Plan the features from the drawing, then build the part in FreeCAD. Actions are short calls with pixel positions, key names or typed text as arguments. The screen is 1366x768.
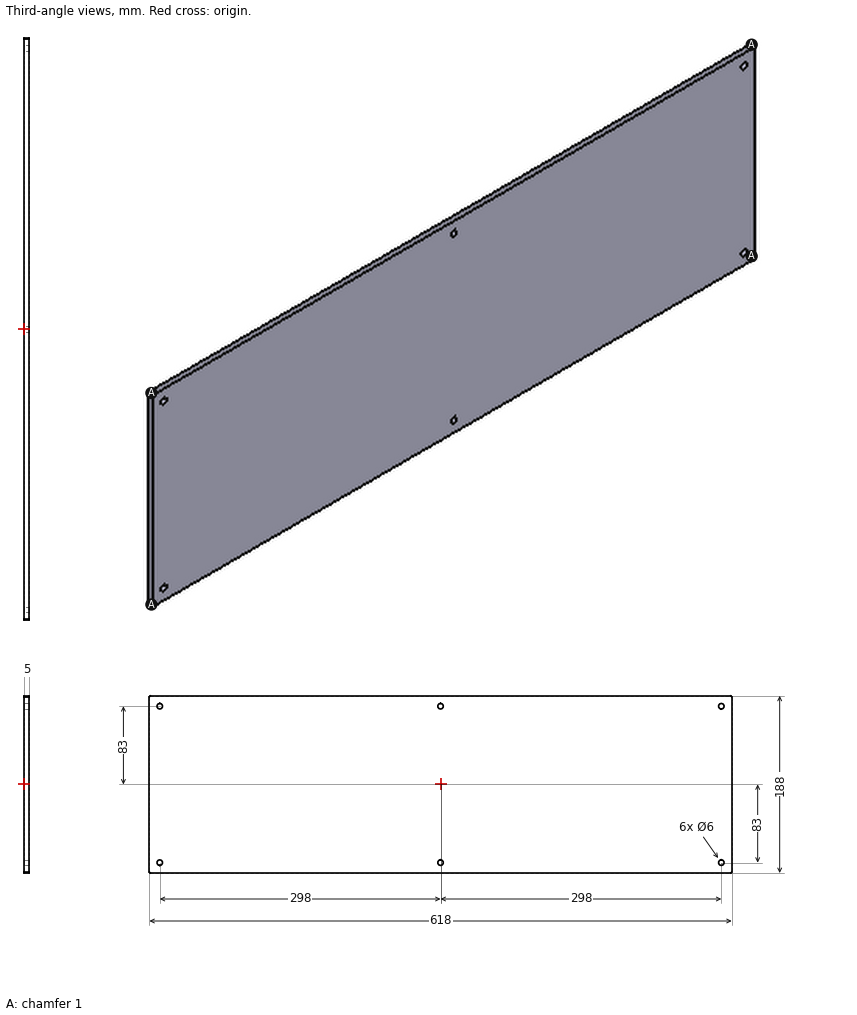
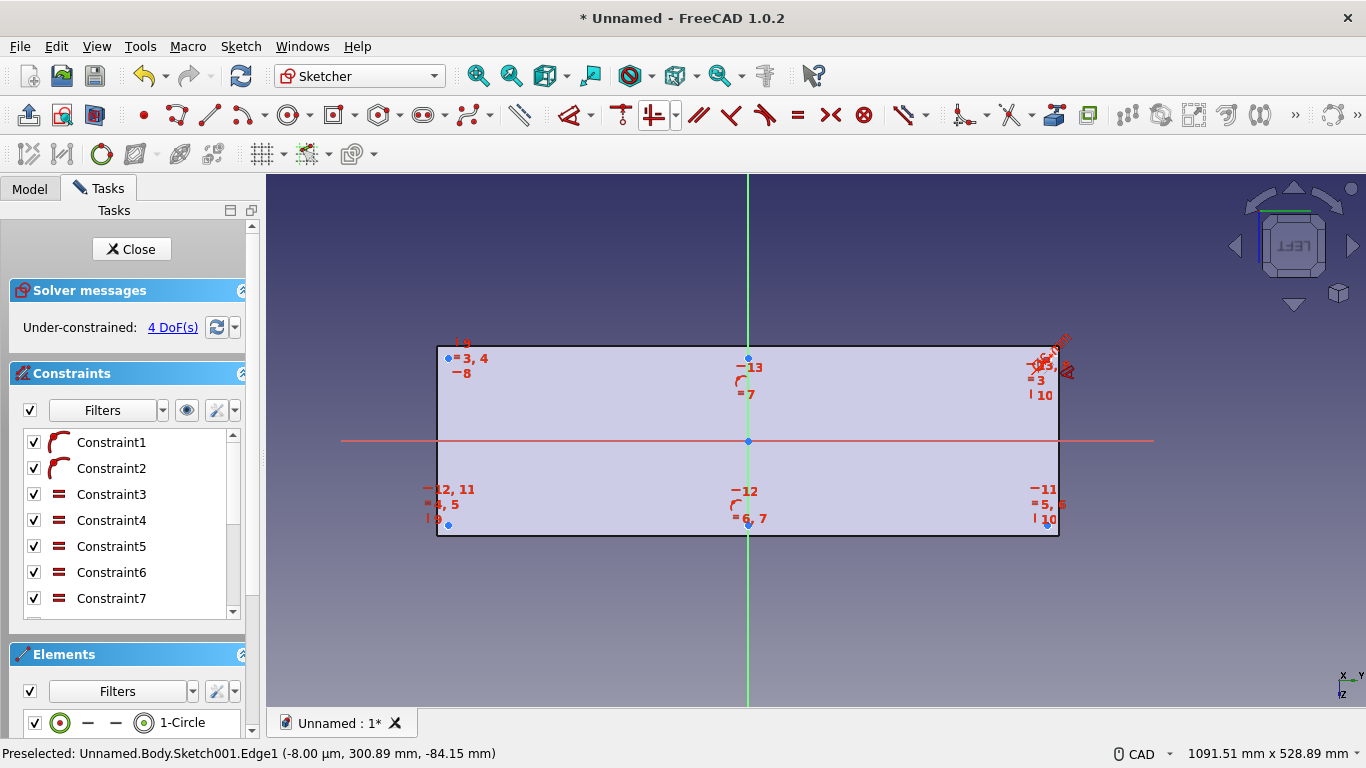
click(1048, 359)
click(1082, 400)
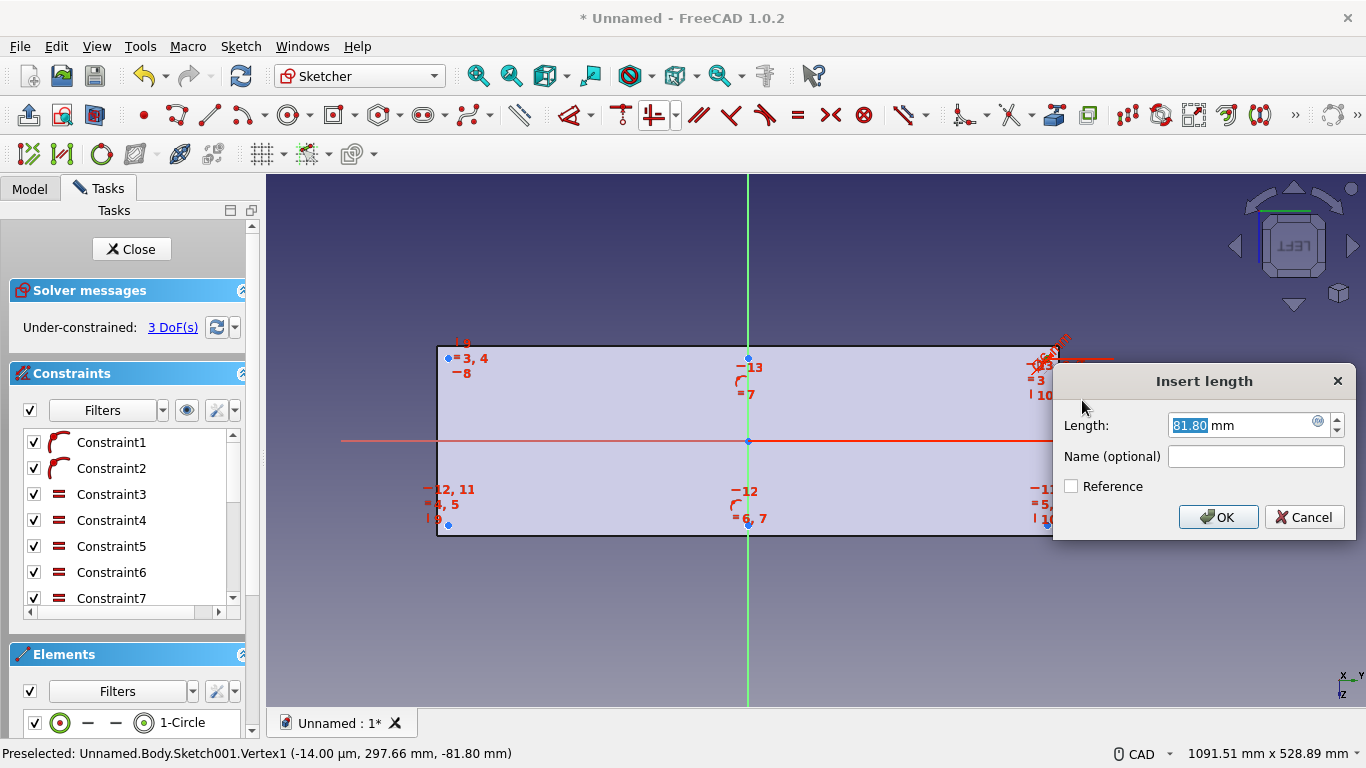
text(83)
key(Return)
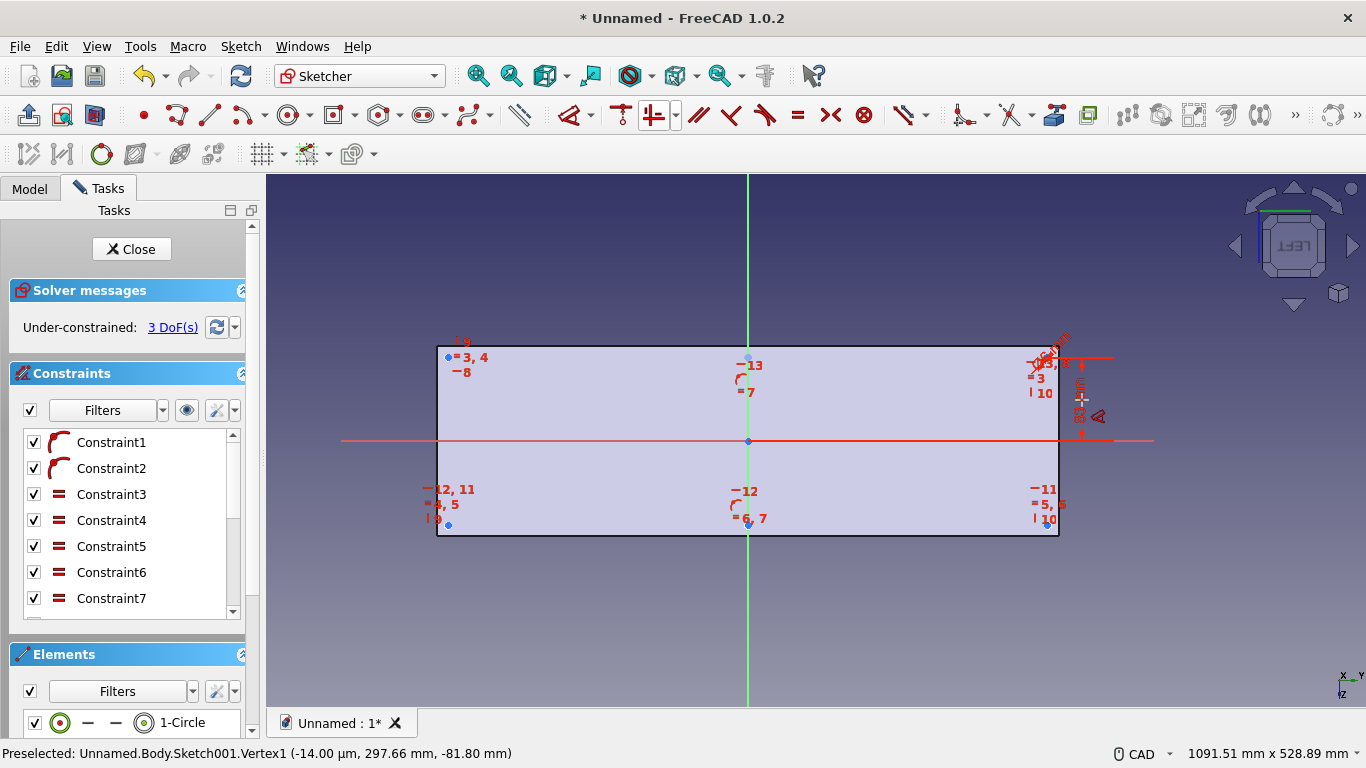
click(448, 526)
click(414, 484)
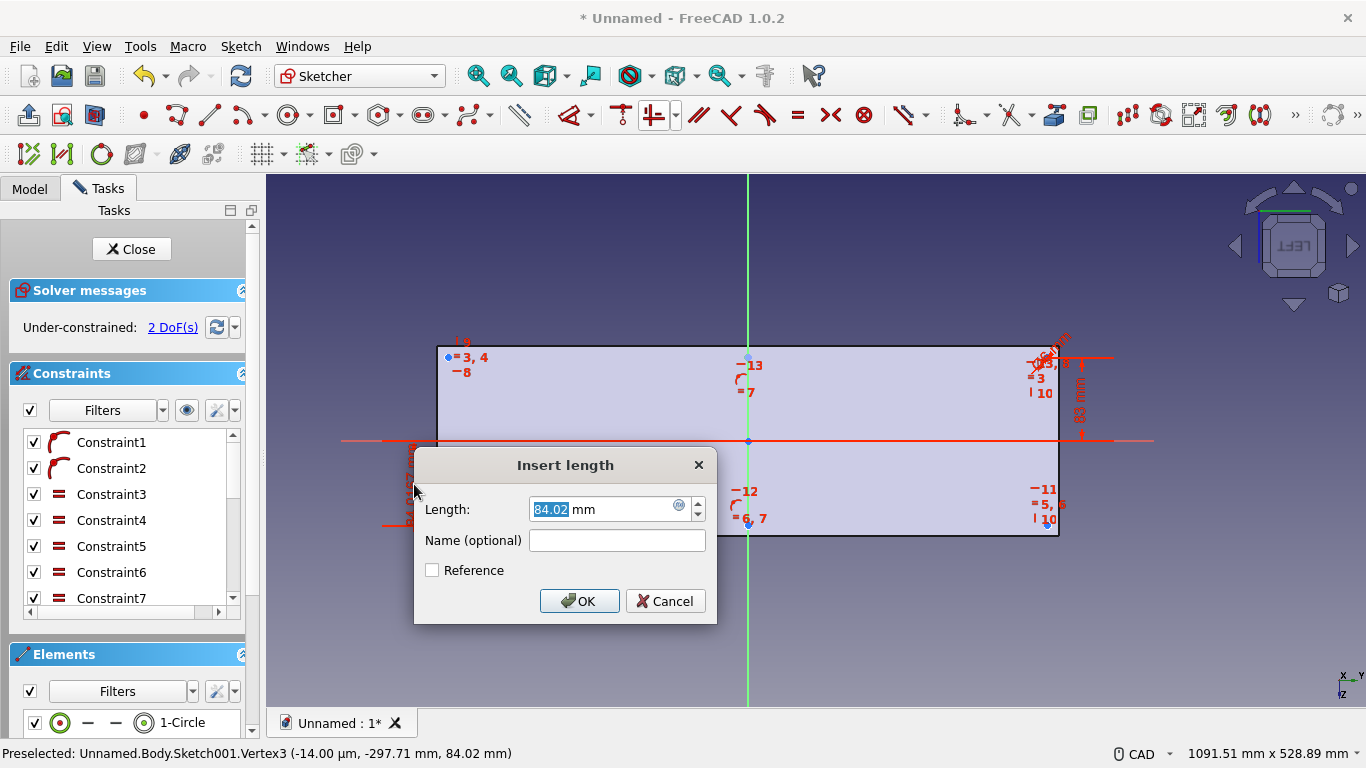
text(83)
key(Return)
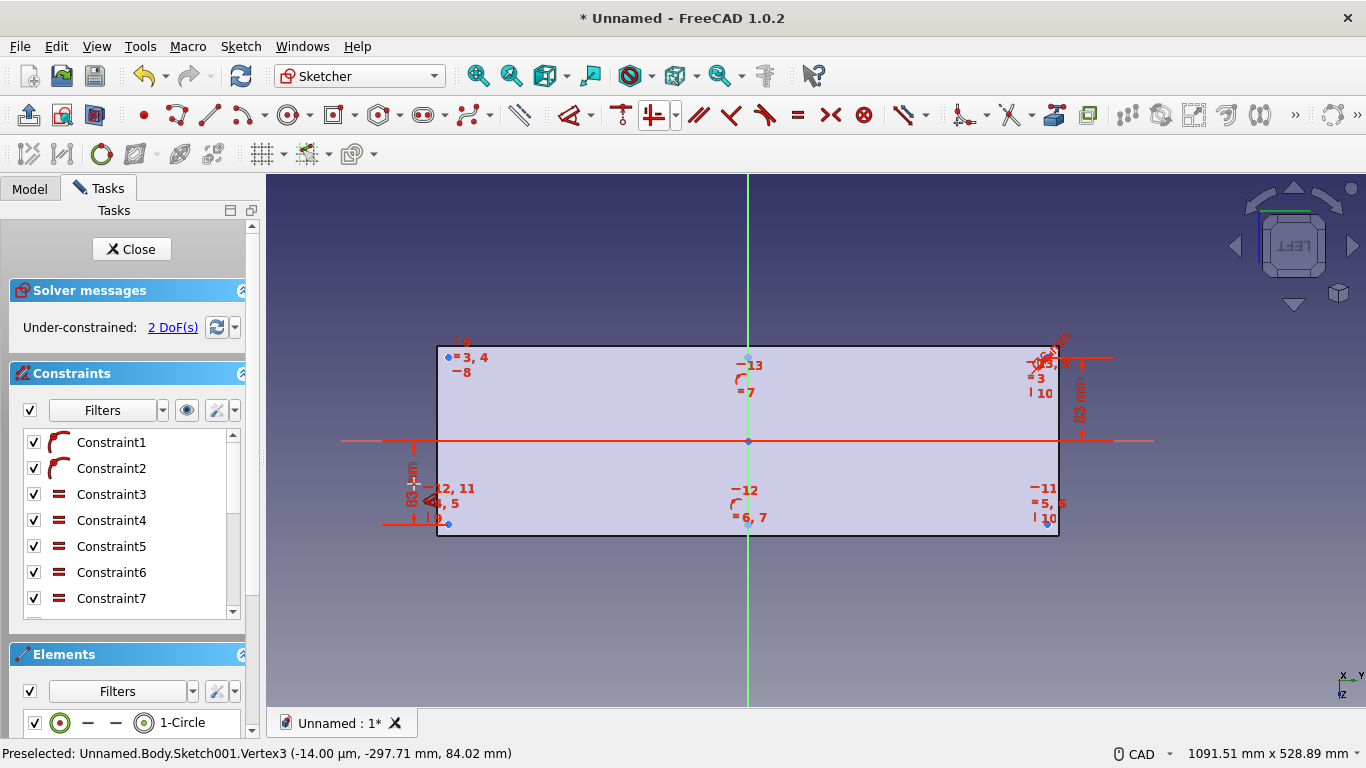
click(1048, 358)
click(898, 324)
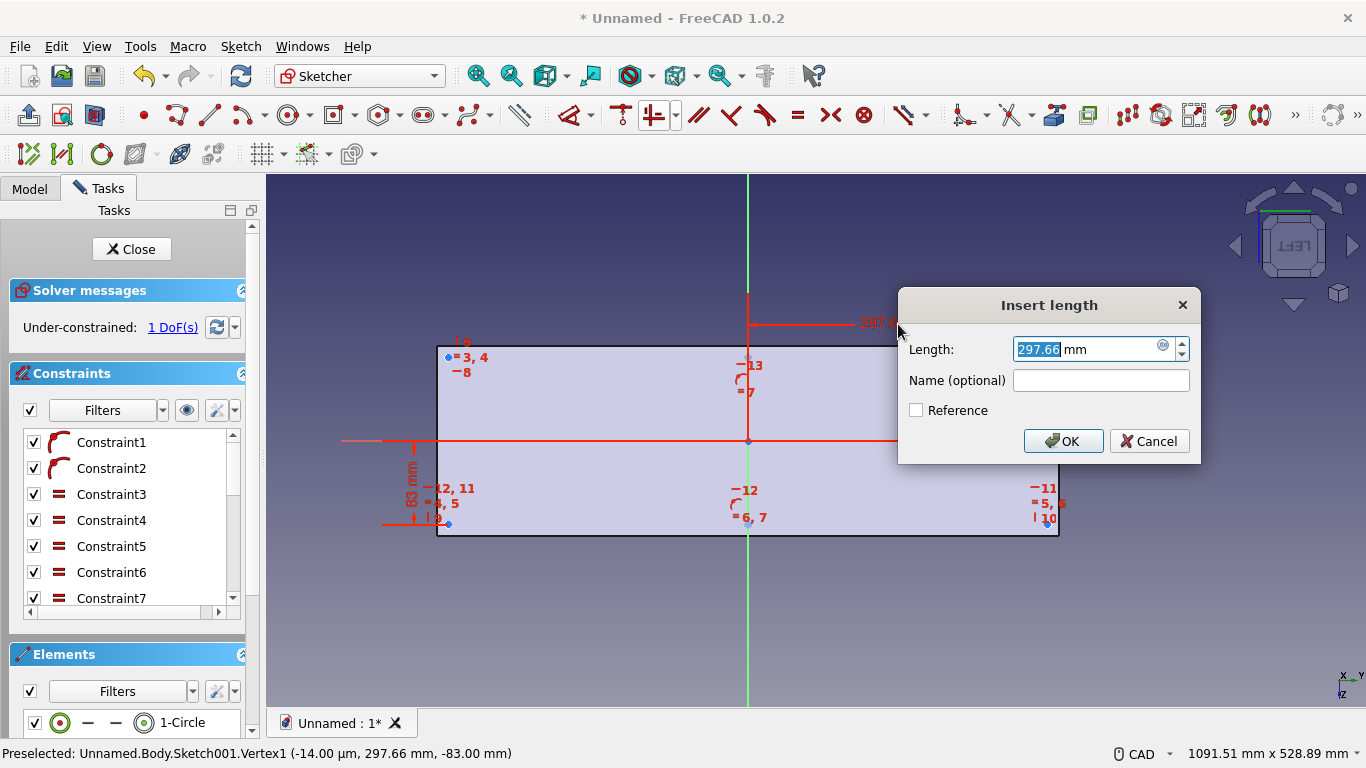
text(298)
key(Return)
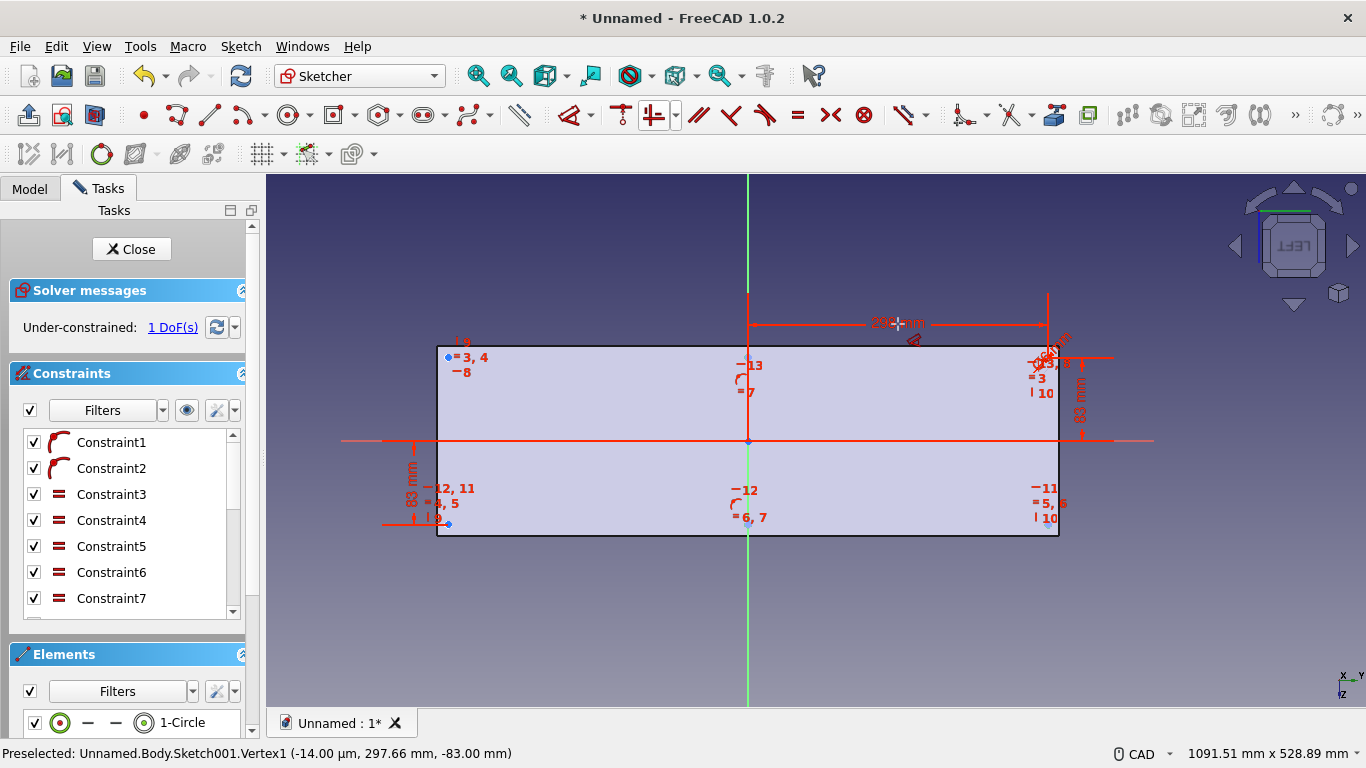
click(448, 358)
click(598, 324)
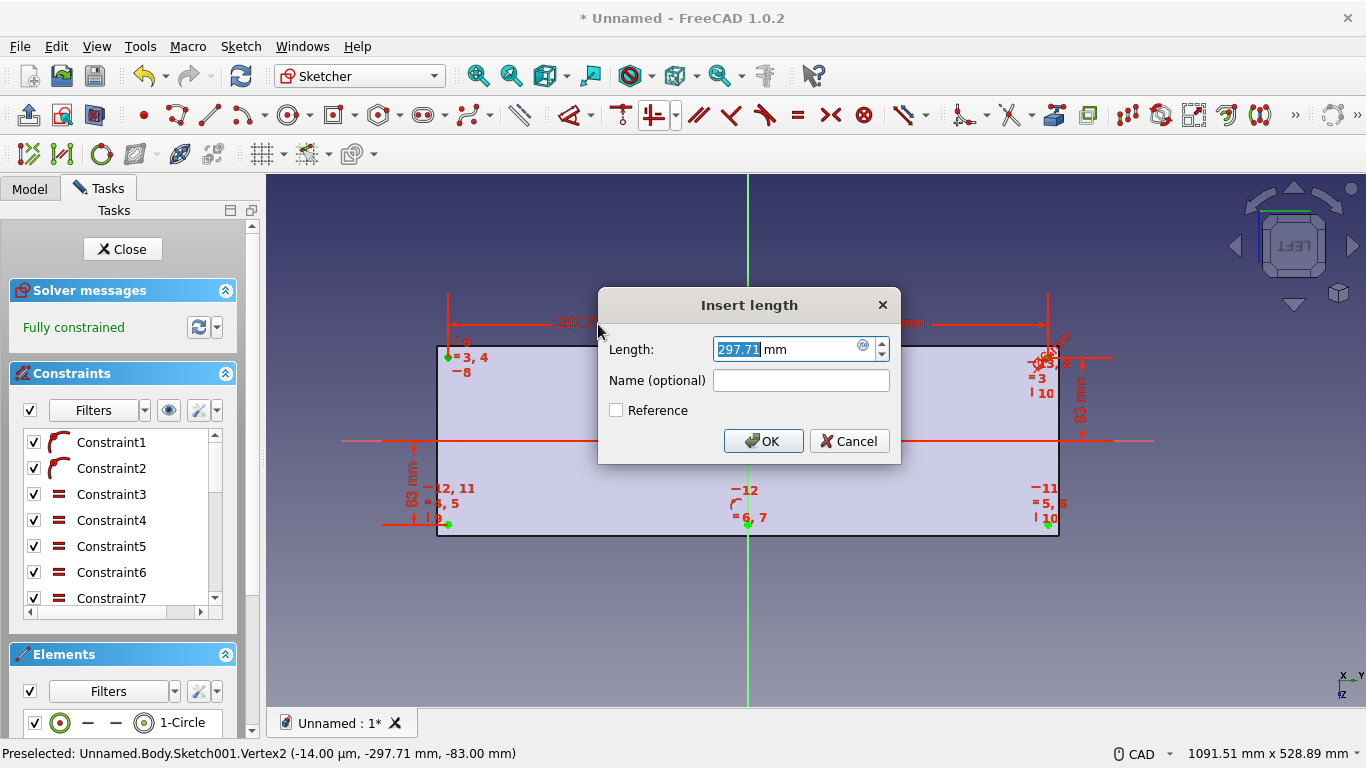
text(298)
key(Return)
key(Escape)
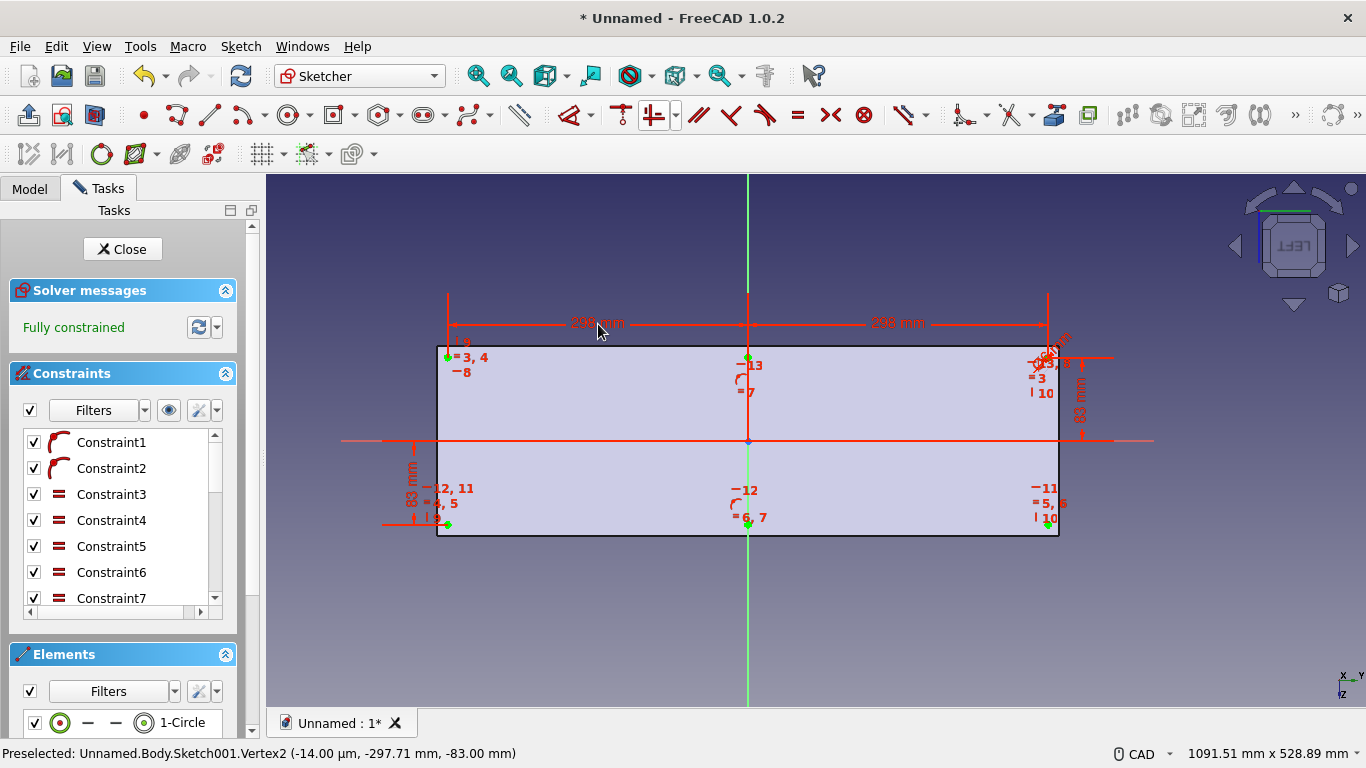
click(123, 249)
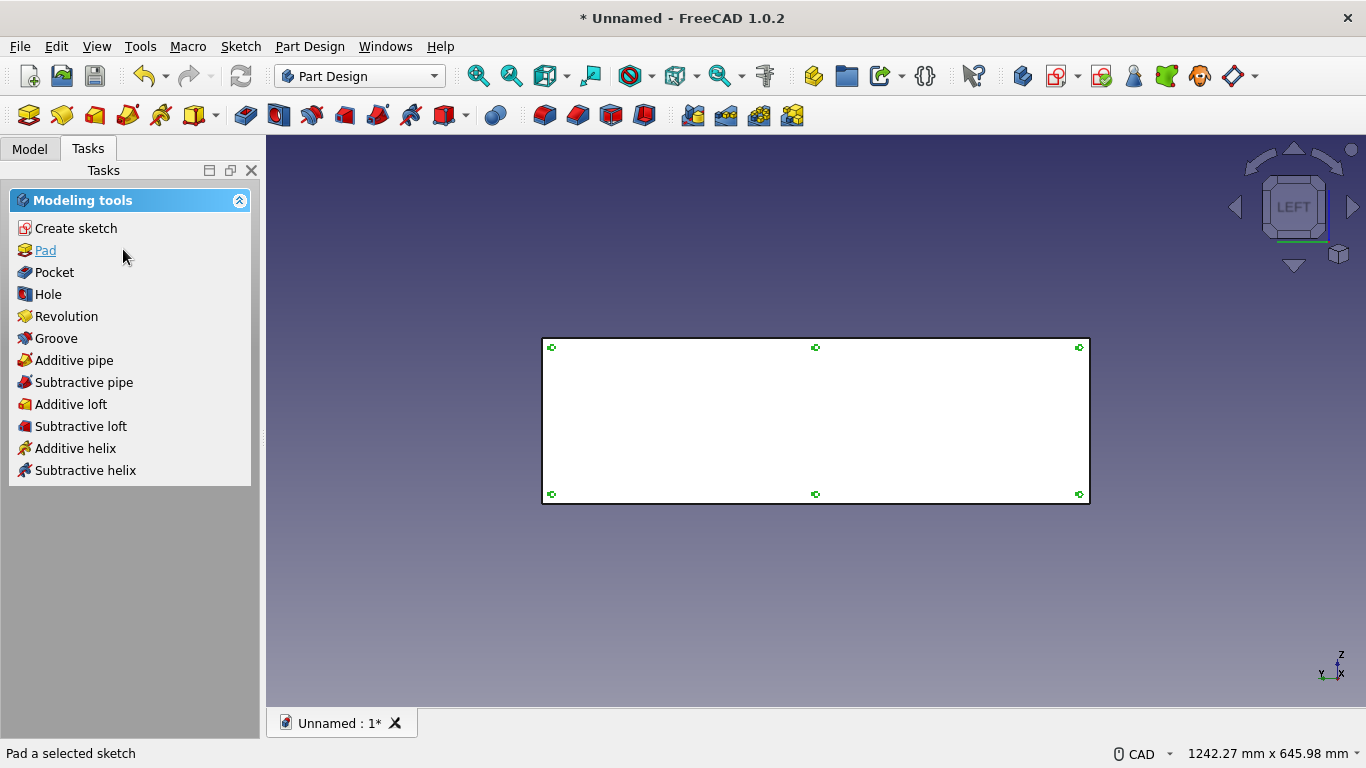
click(246, 116)